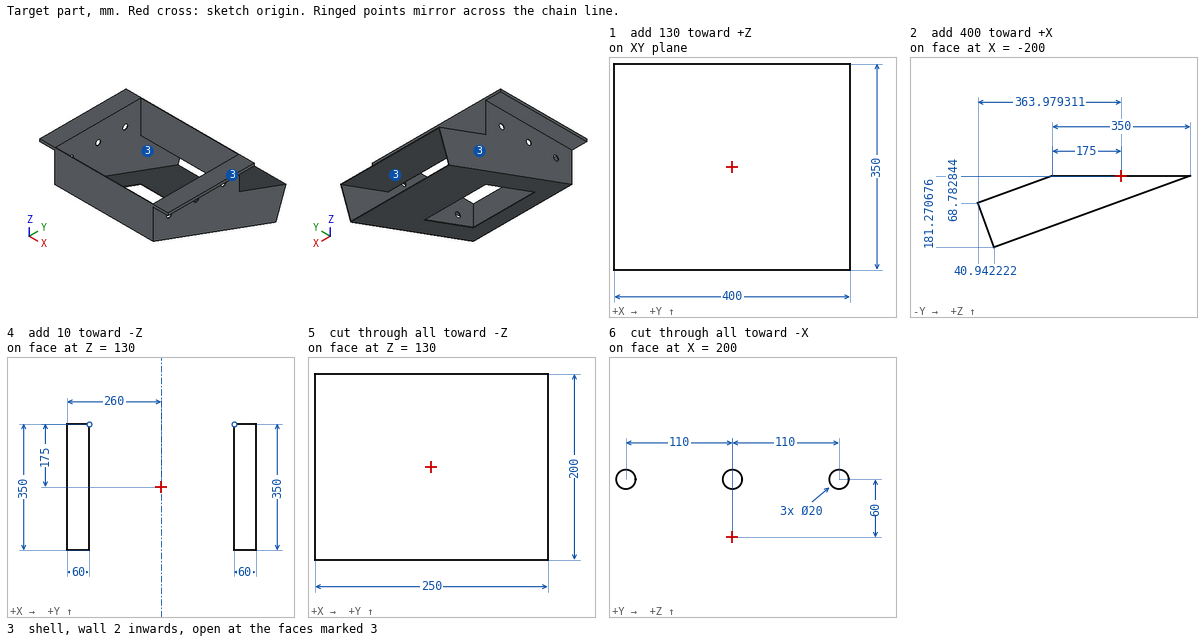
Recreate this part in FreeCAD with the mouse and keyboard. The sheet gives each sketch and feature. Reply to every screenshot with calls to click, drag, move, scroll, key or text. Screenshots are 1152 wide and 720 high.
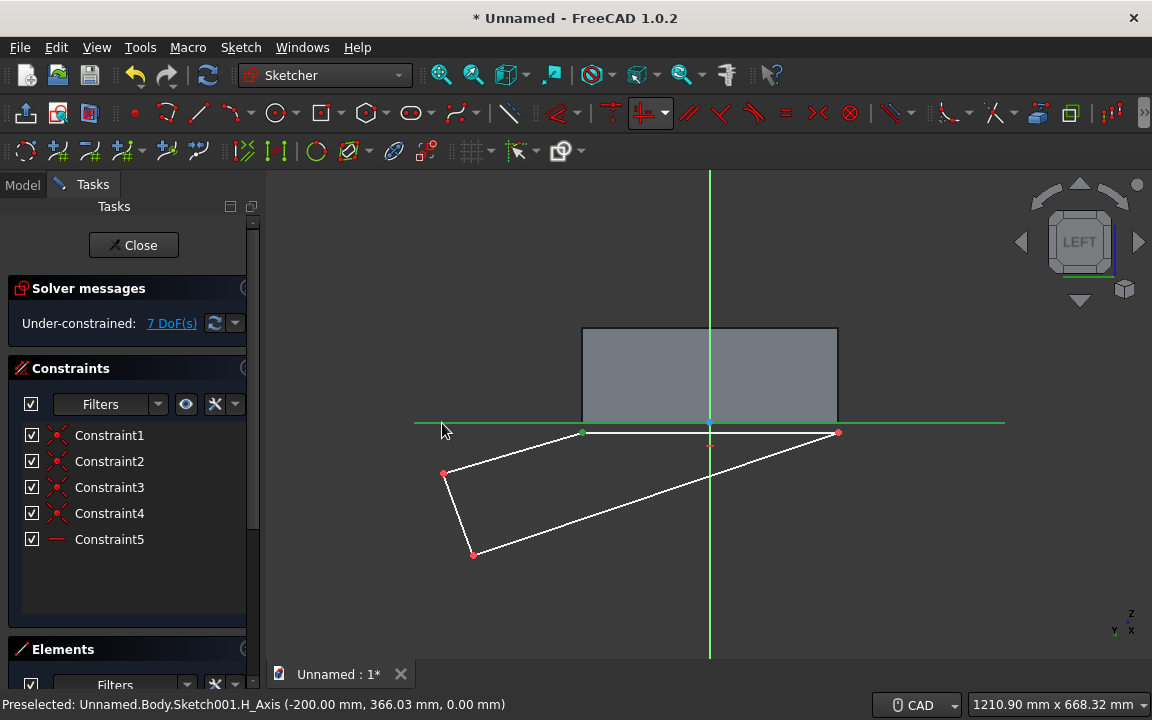
click(612, 114)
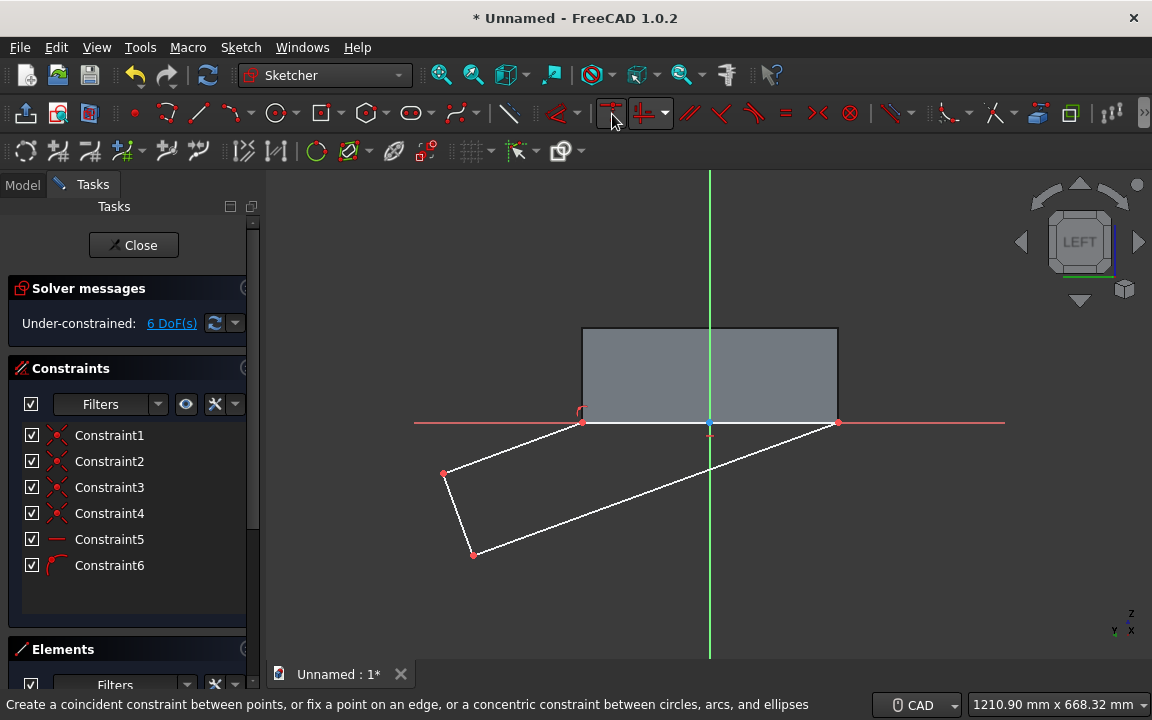
click(761, 423)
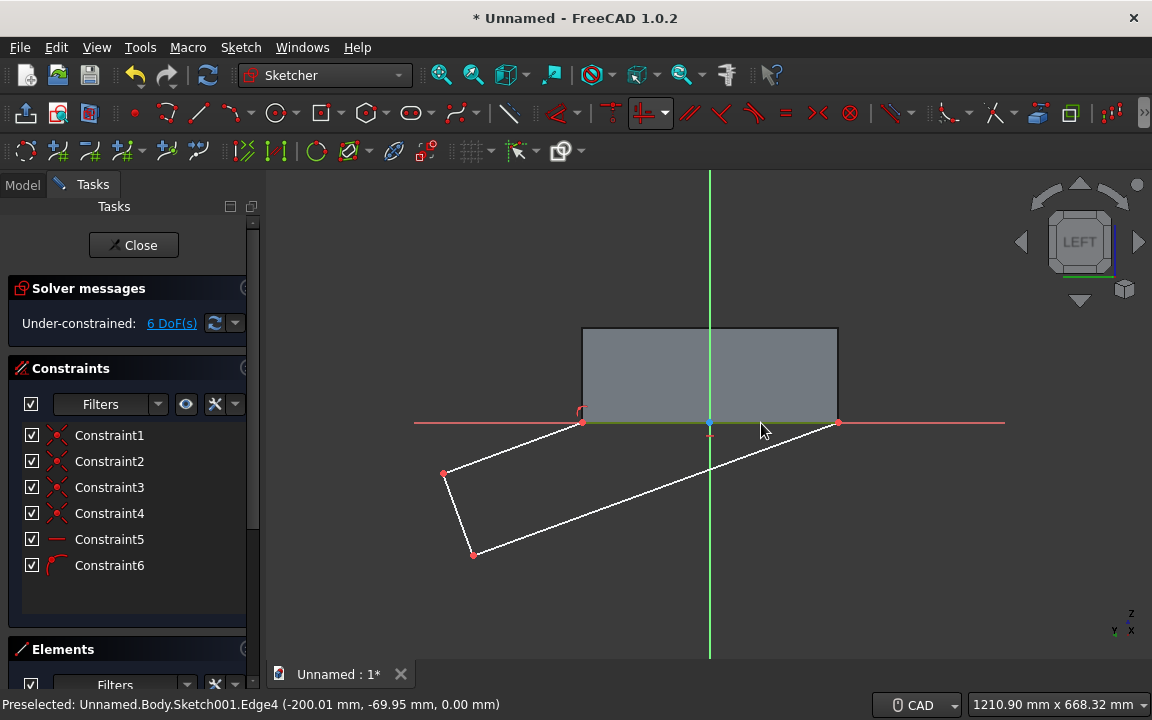
key(l)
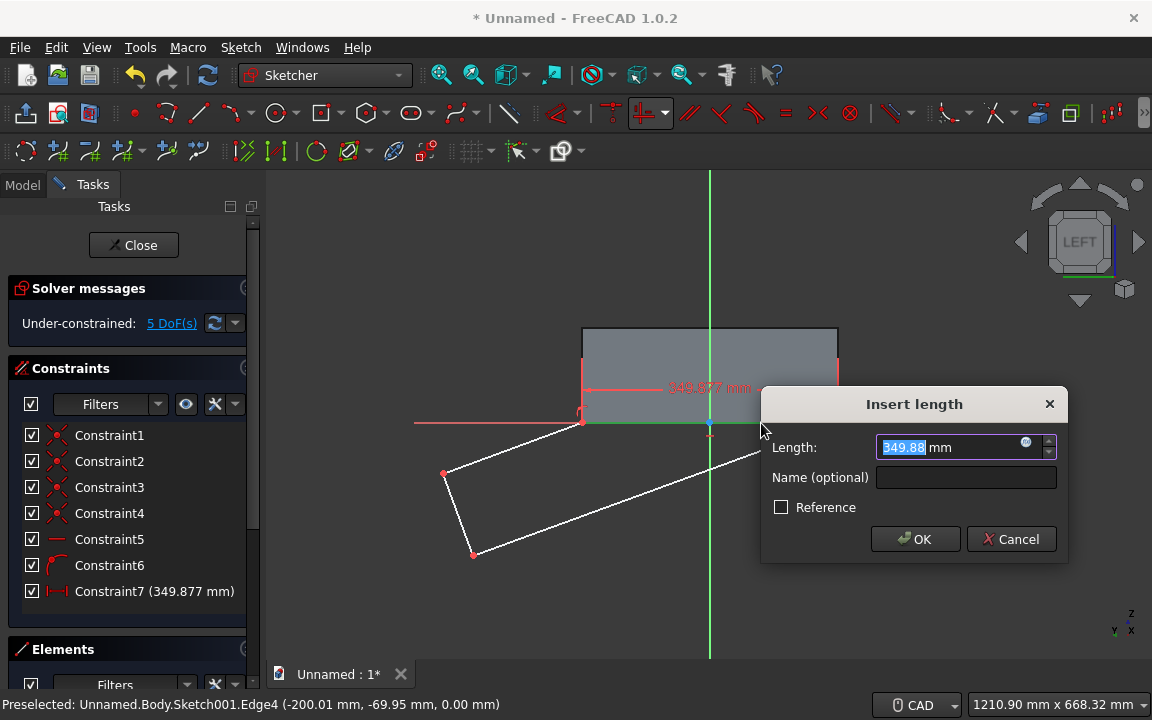
text(350)
key(Return)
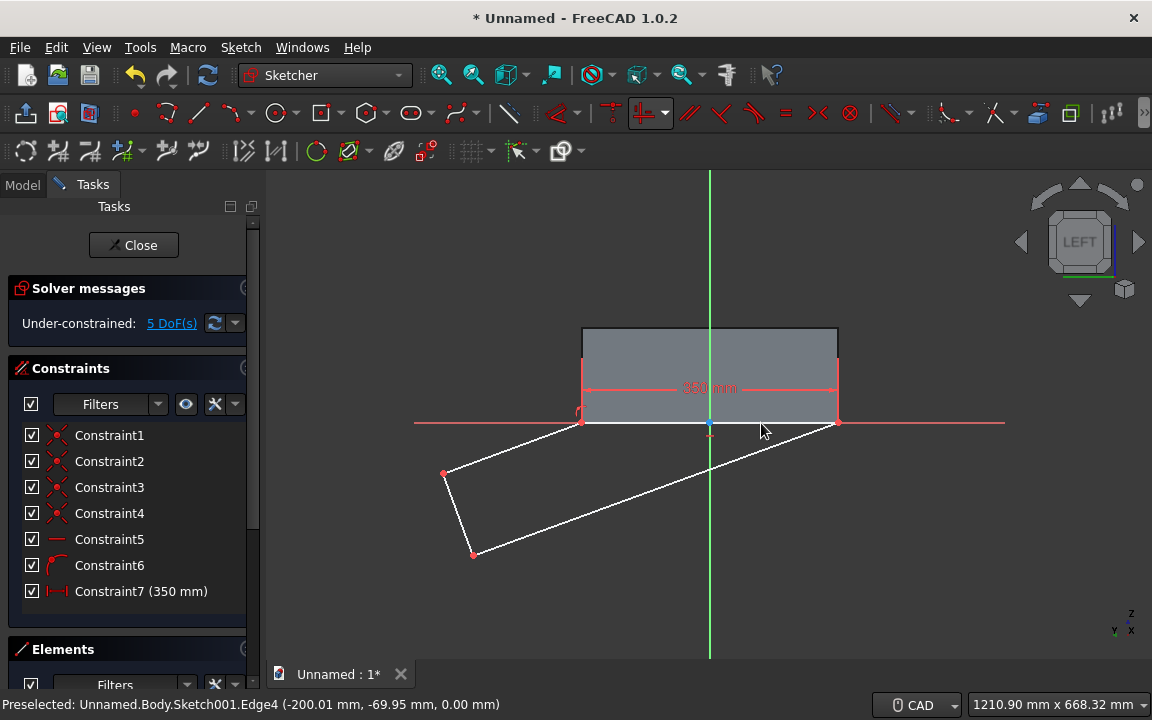
click(582, 423)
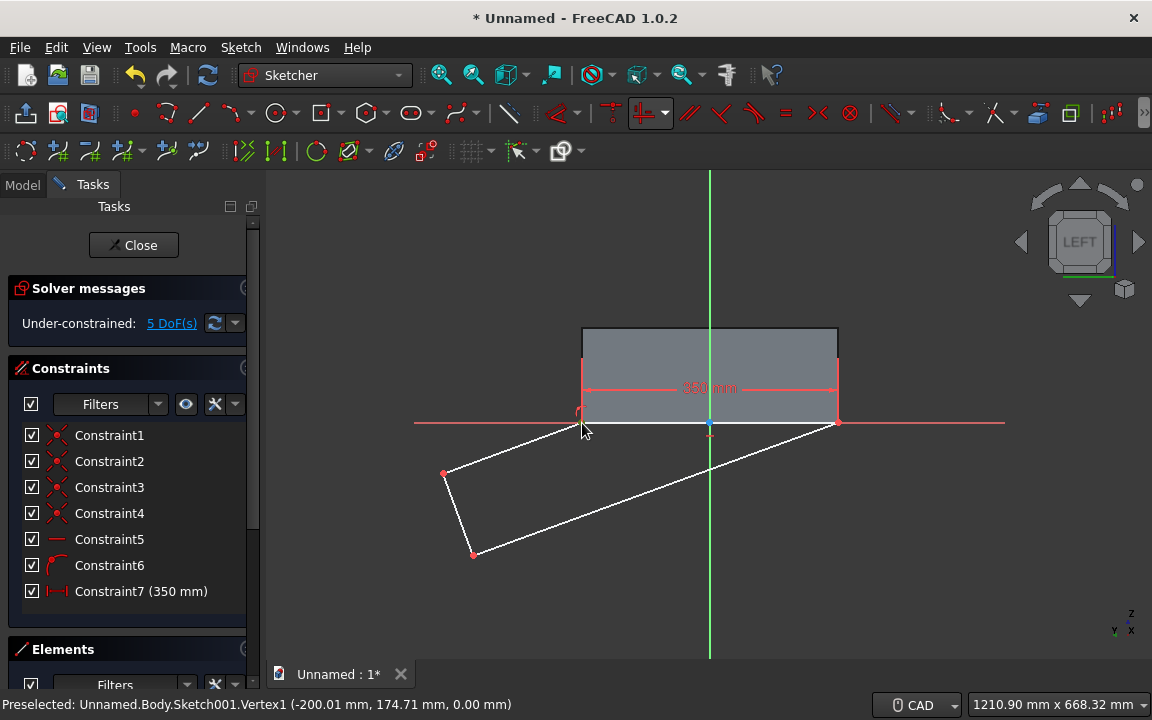
key(l)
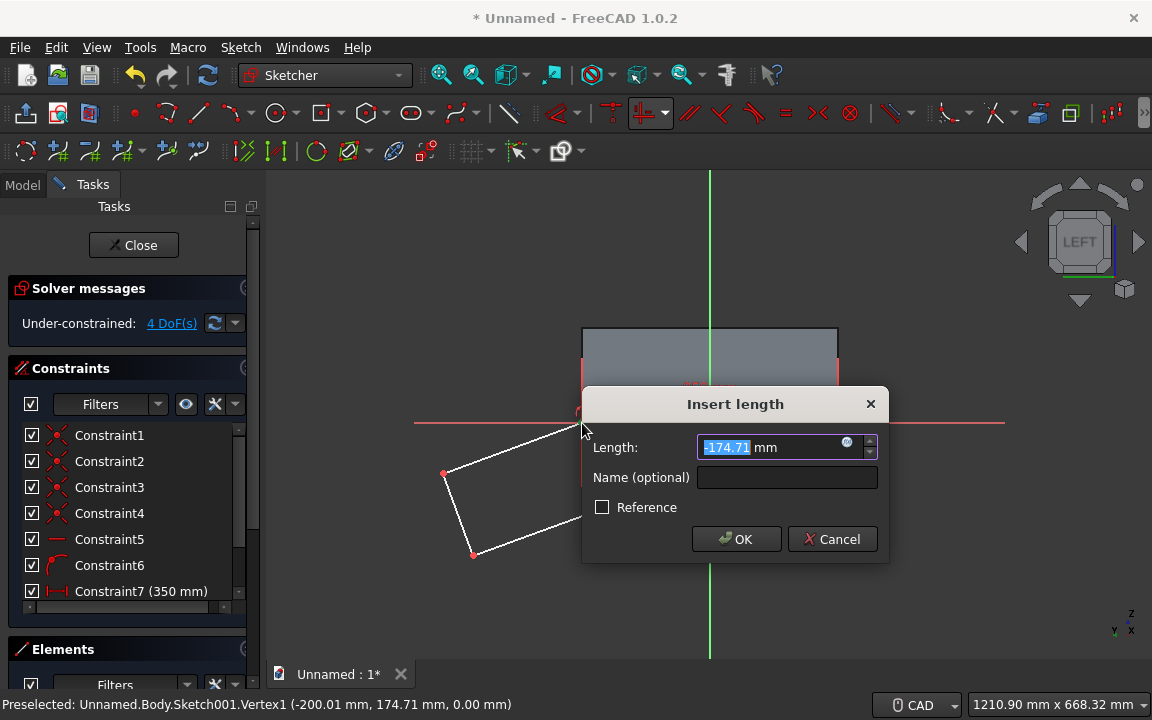
text(-175)
key(Return)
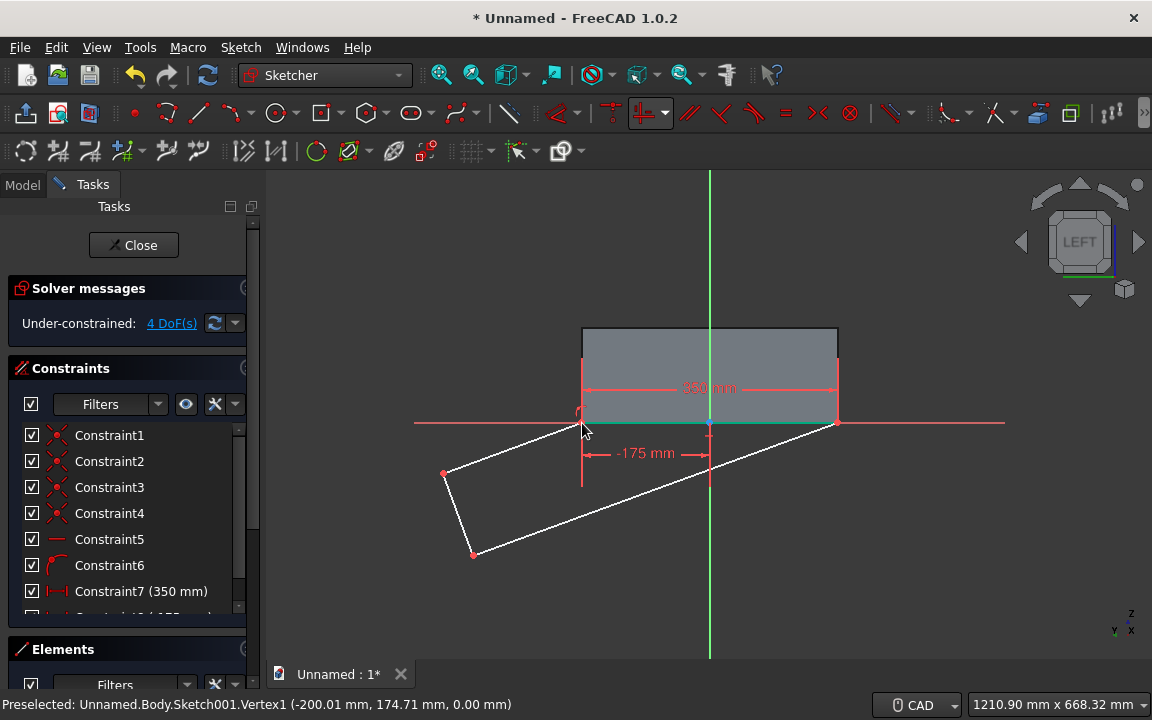
click(443, 474)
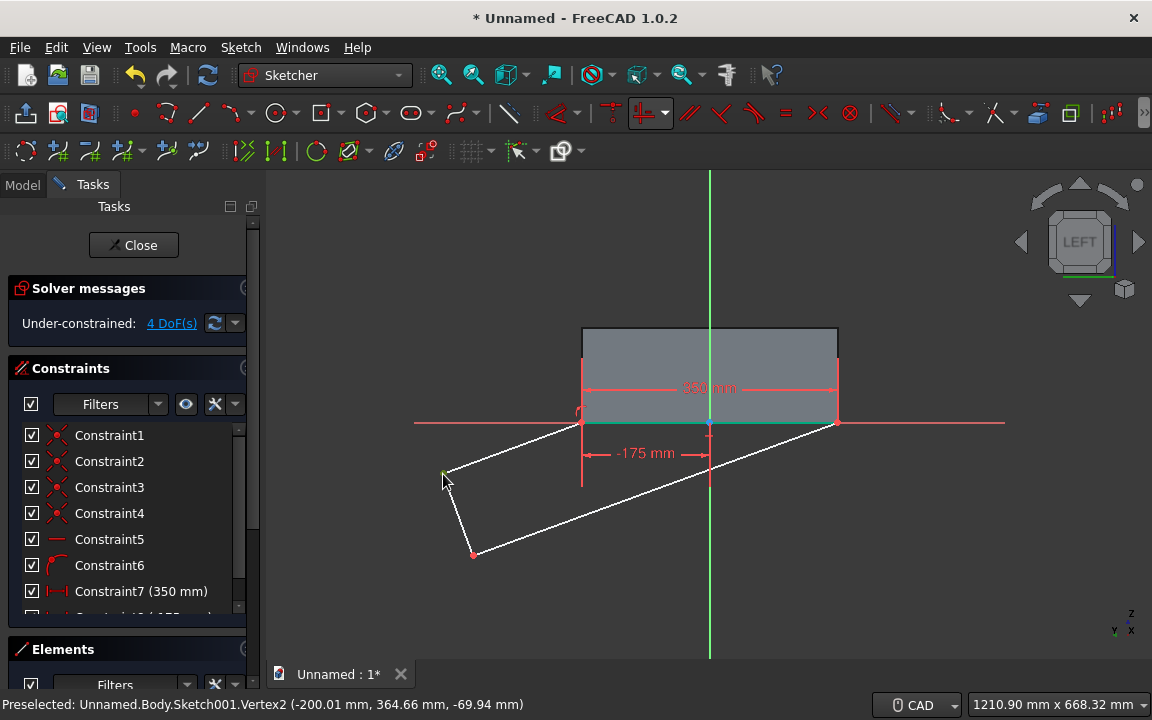
key(i)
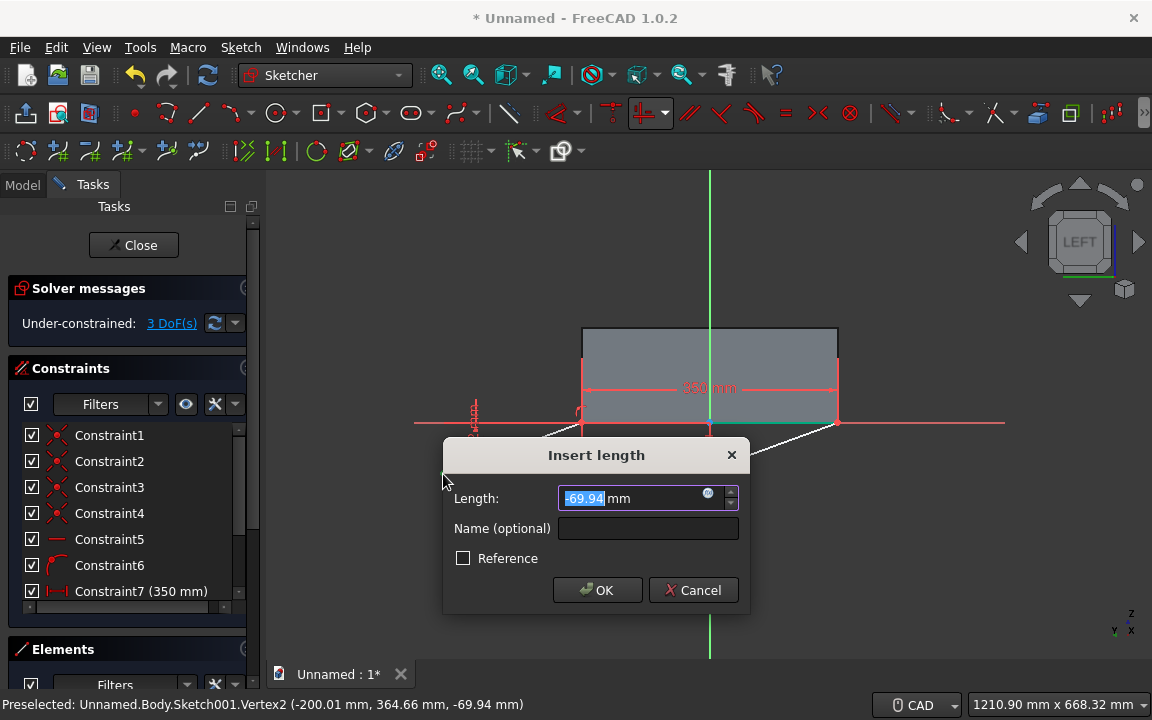
text(-68.782844)
key(Return)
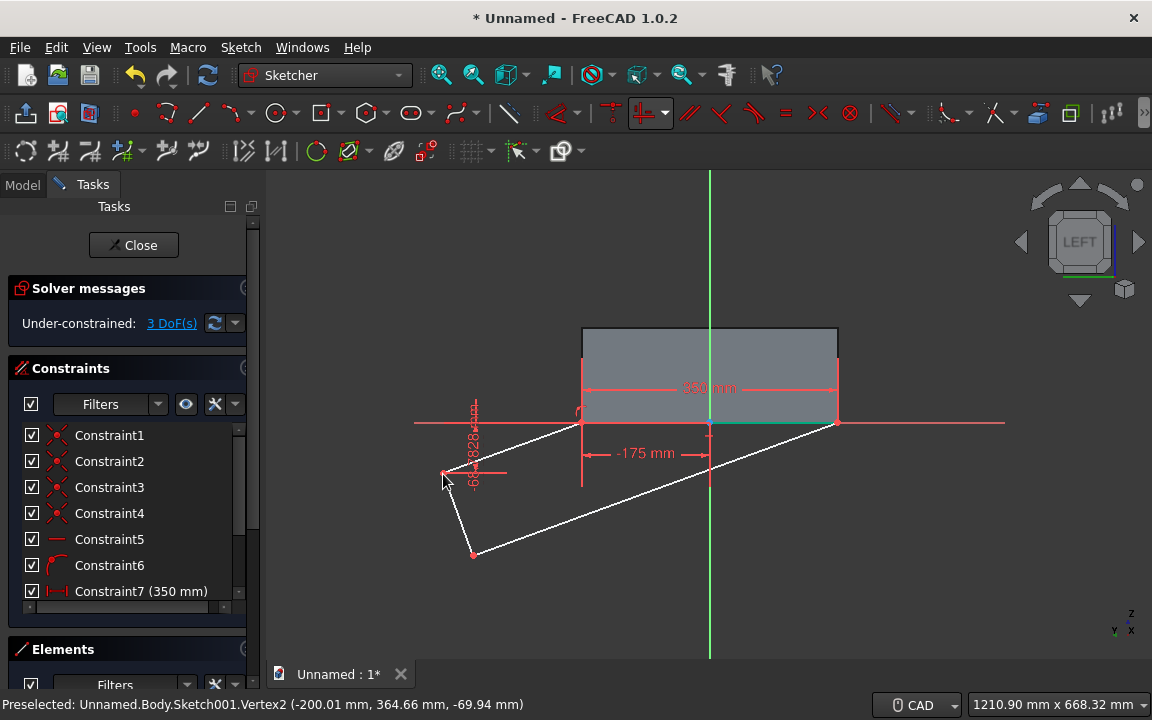
scroll(452, 498, up, 2)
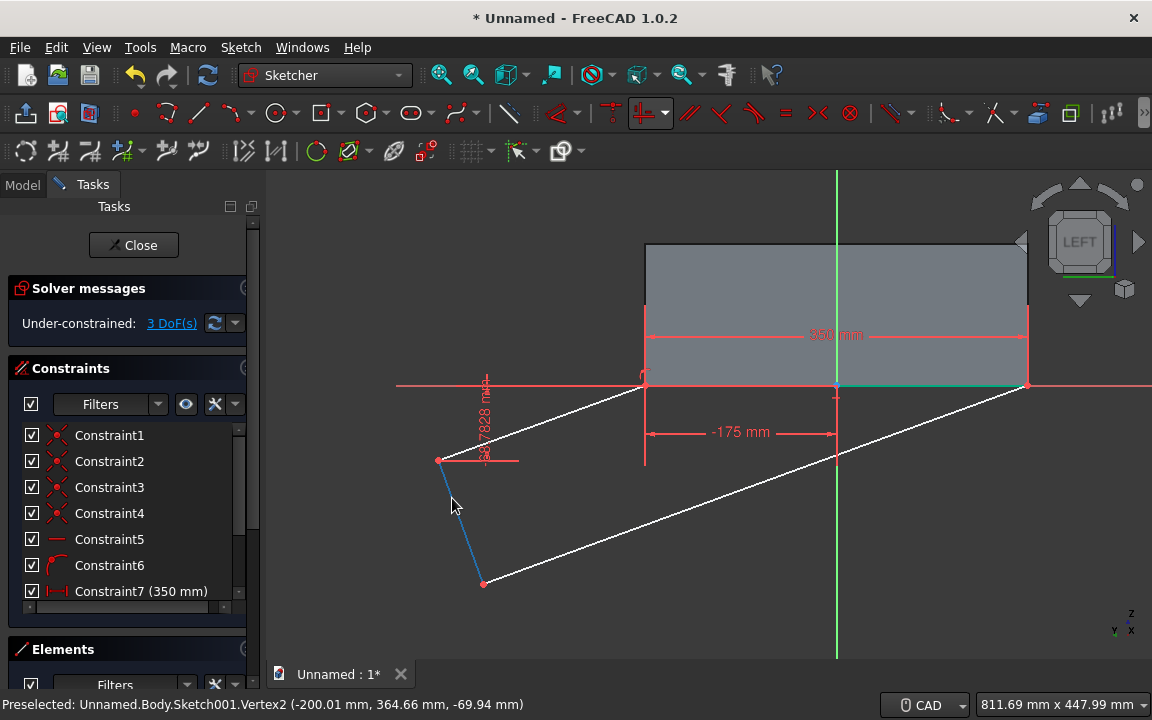
click(452, 498)